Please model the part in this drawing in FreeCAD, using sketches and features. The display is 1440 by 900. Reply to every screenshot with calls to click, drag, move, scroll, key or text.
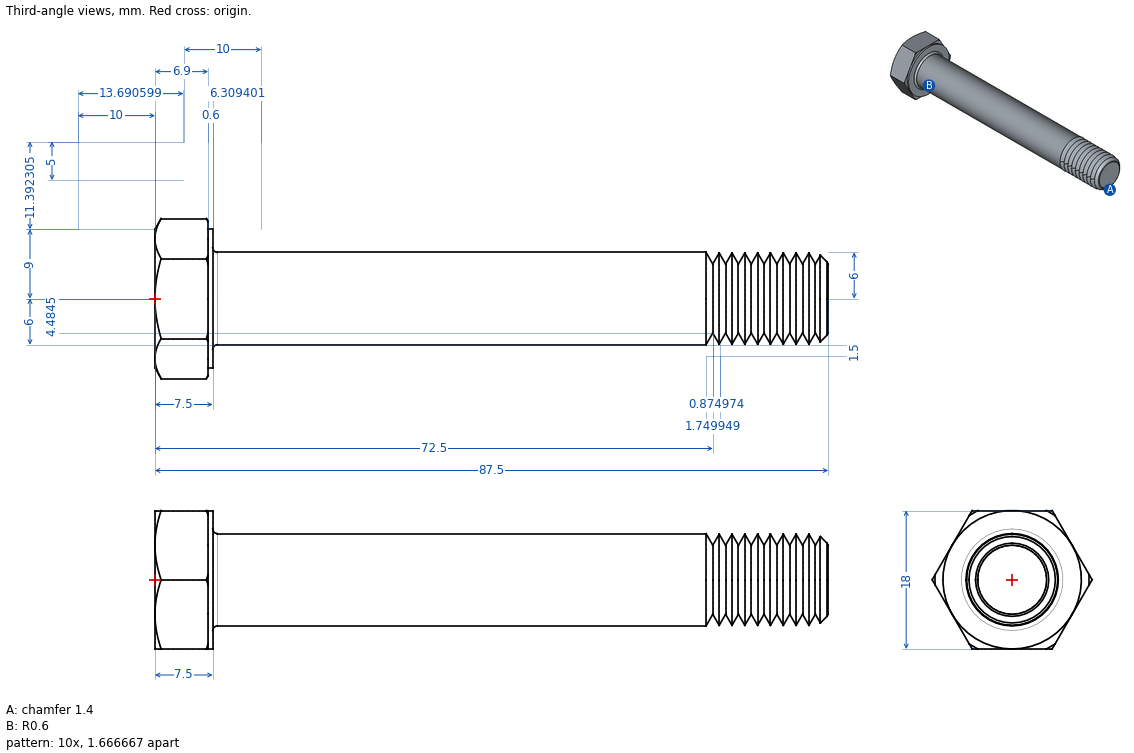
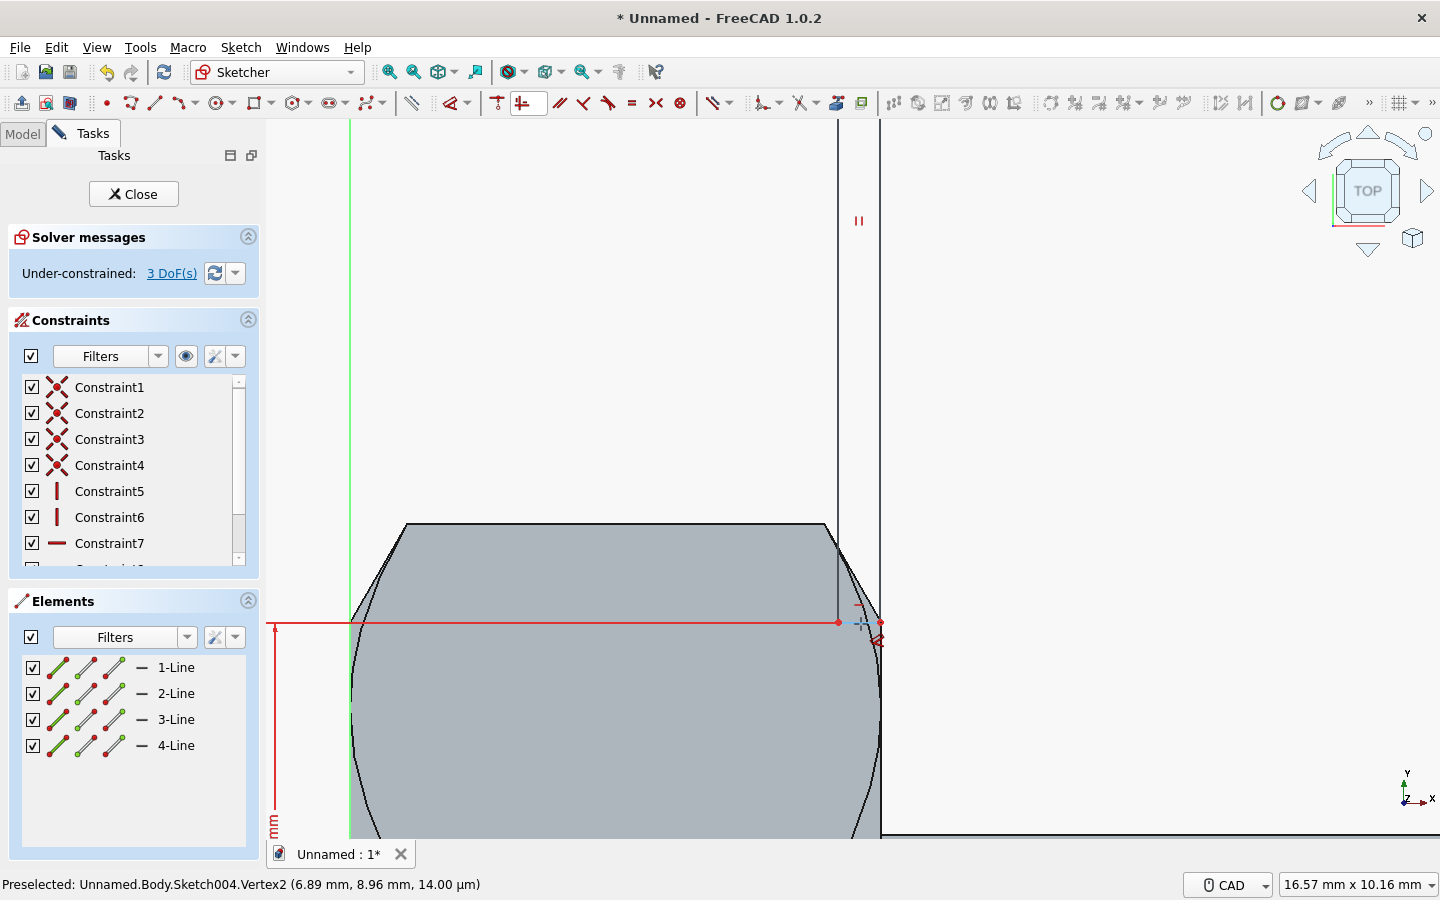
click(859, 623)
click(859, 657)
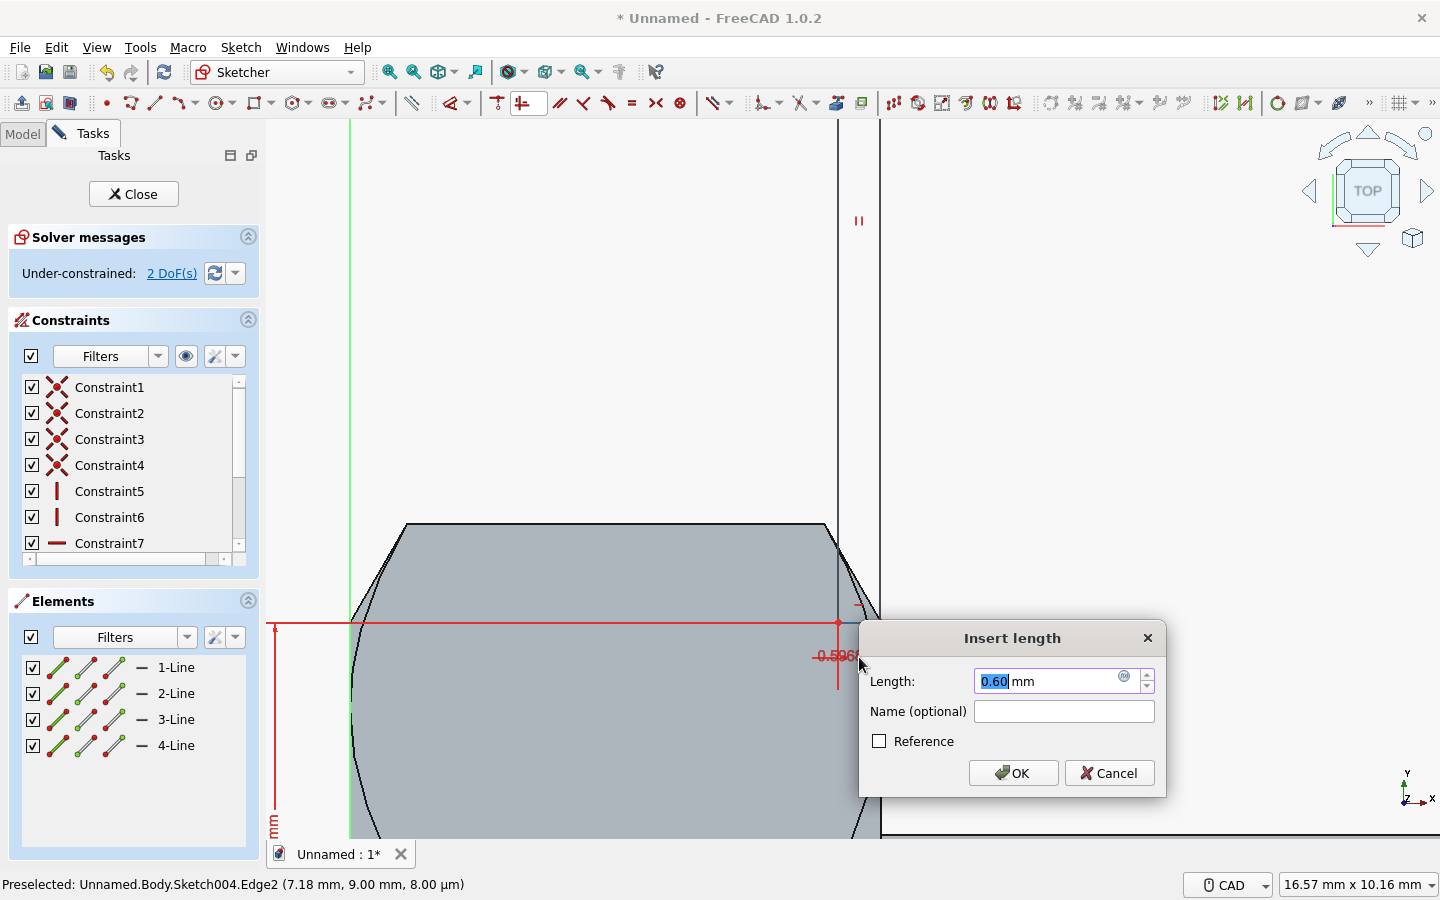
text(0.6)
key(Return)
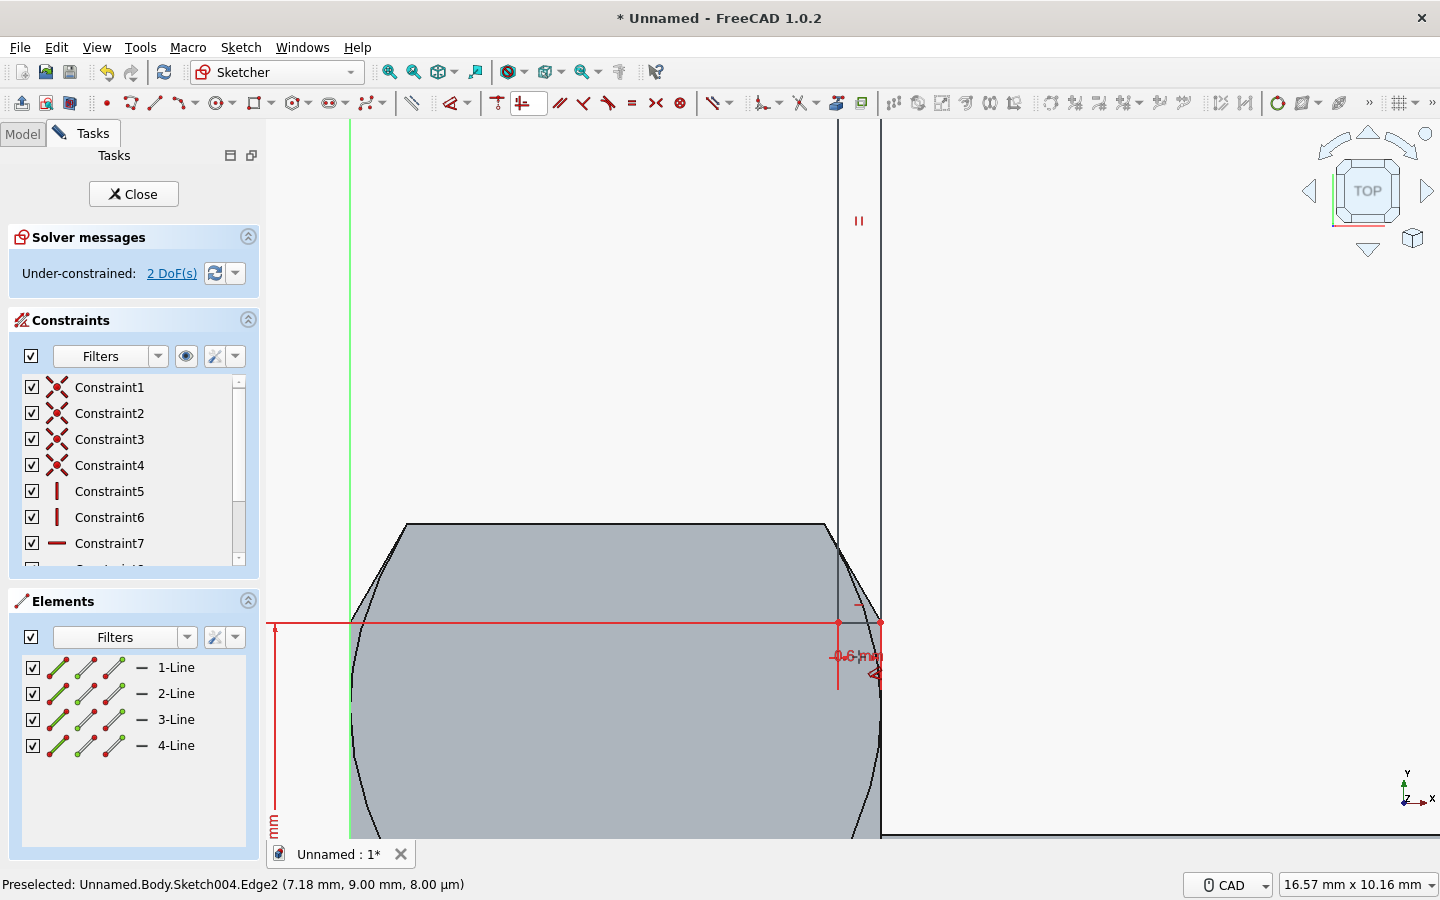
scroll(857, 454, down, 6)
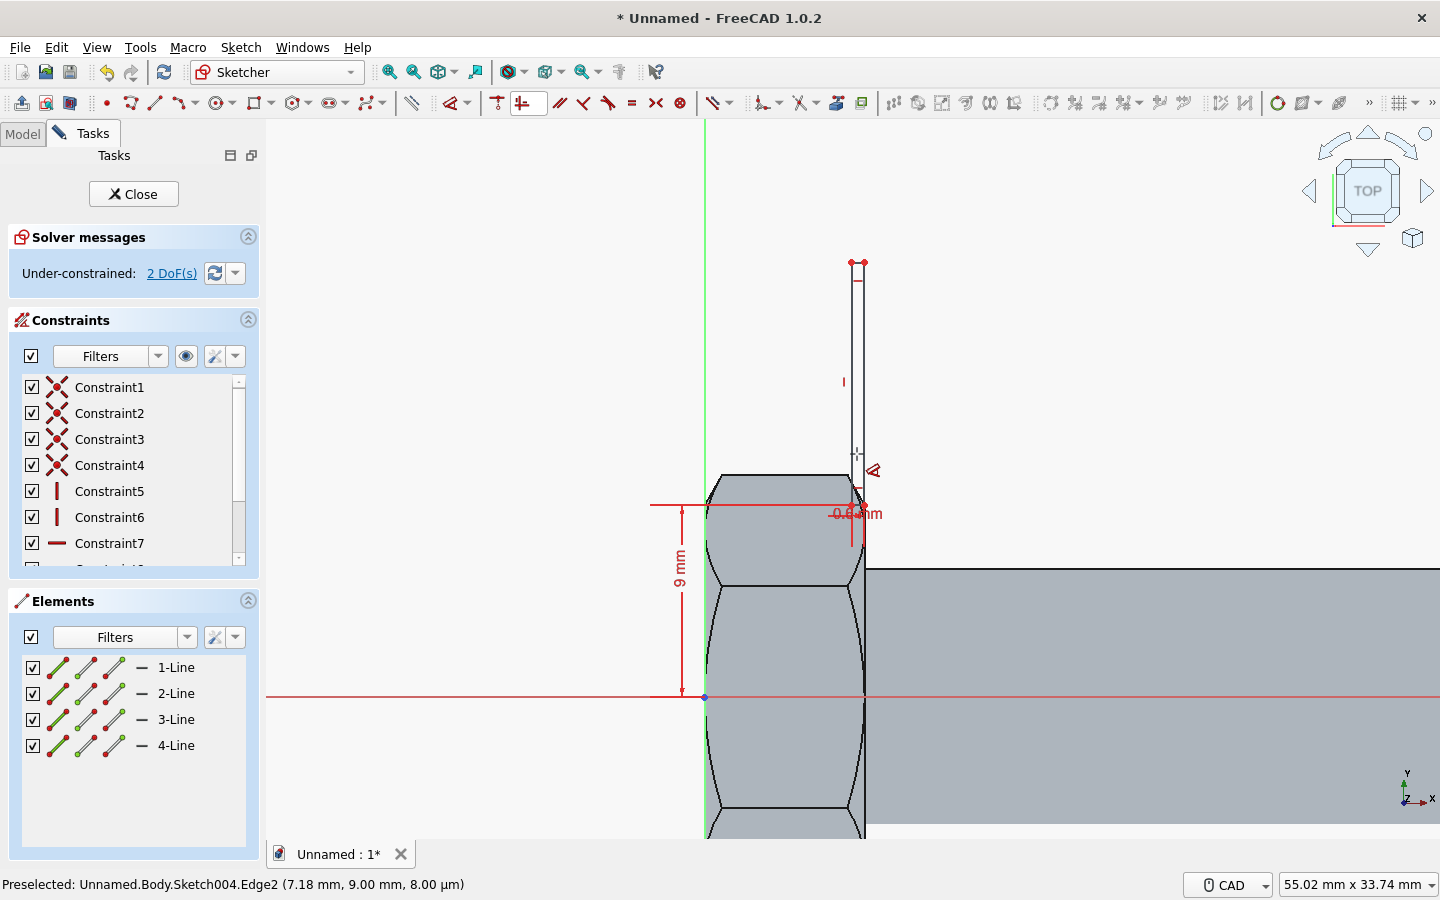
click(852, 263)
click(778, 731)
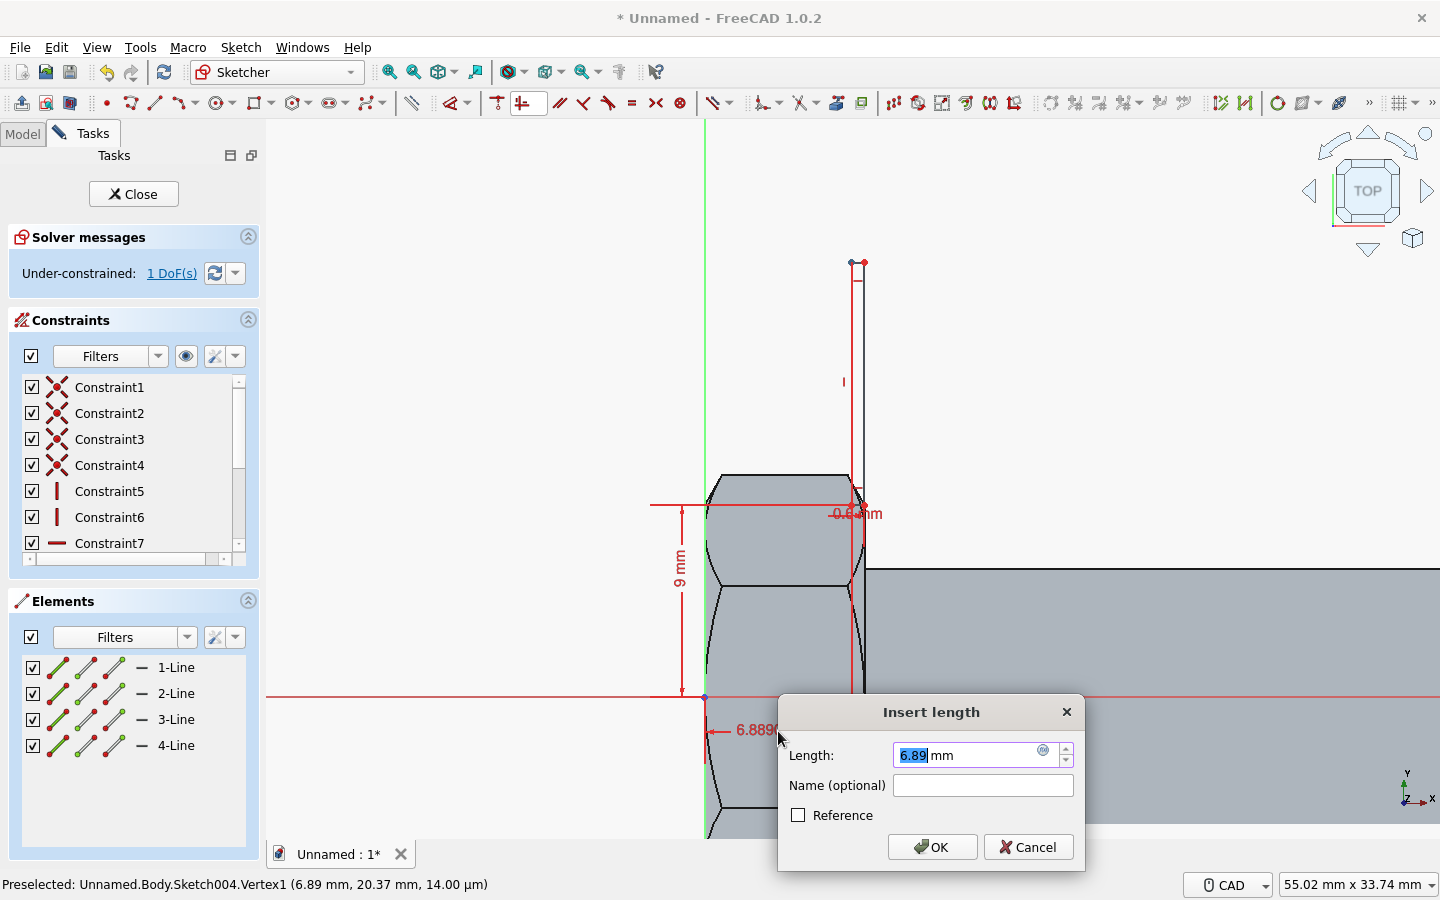
text(6.9)
key(Return)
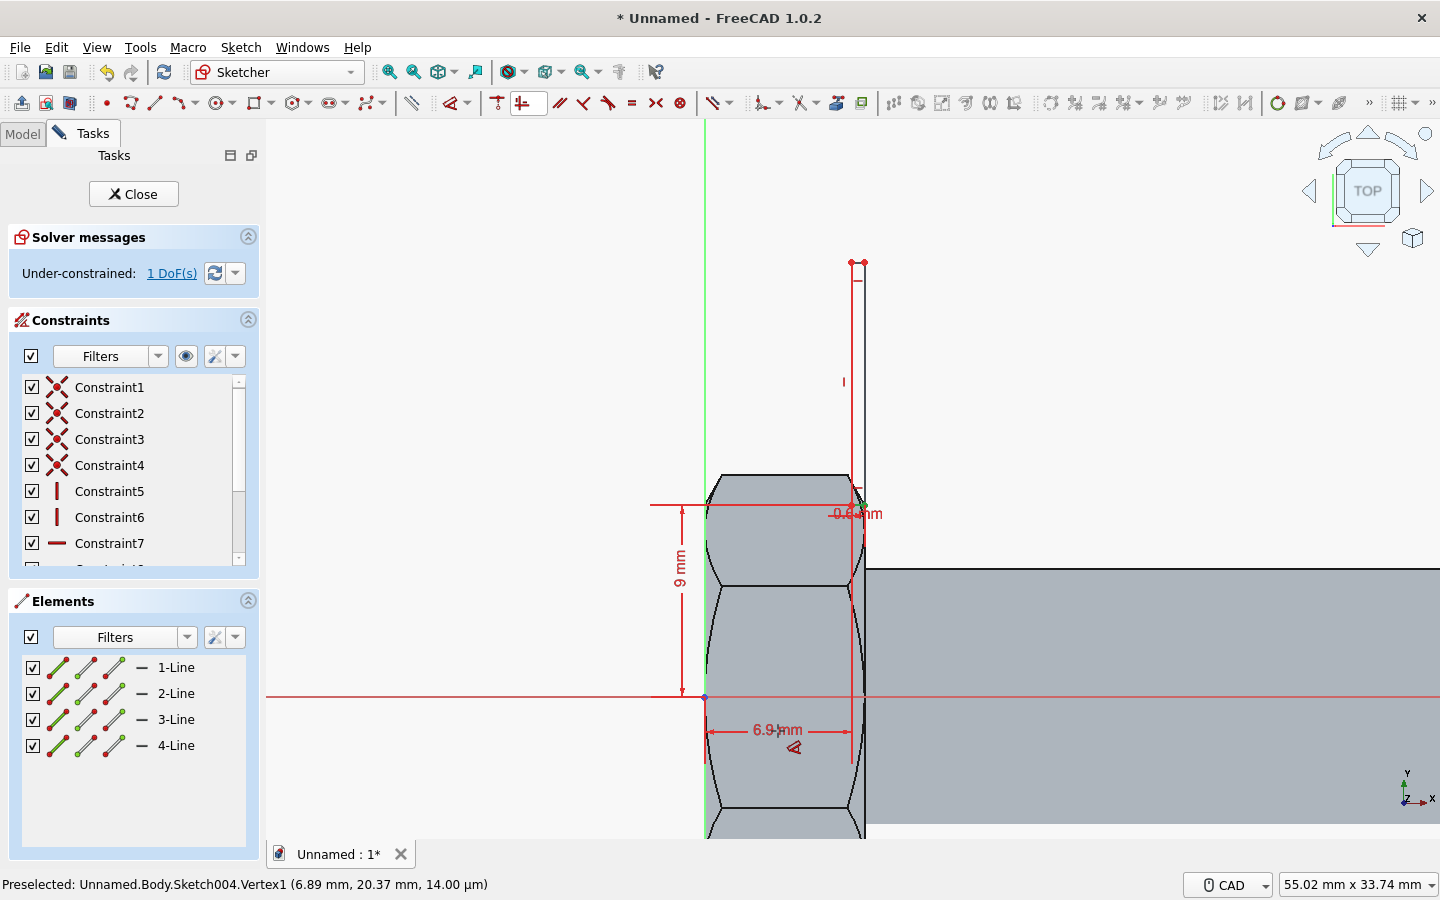
click(852, 335)
click(886, 384)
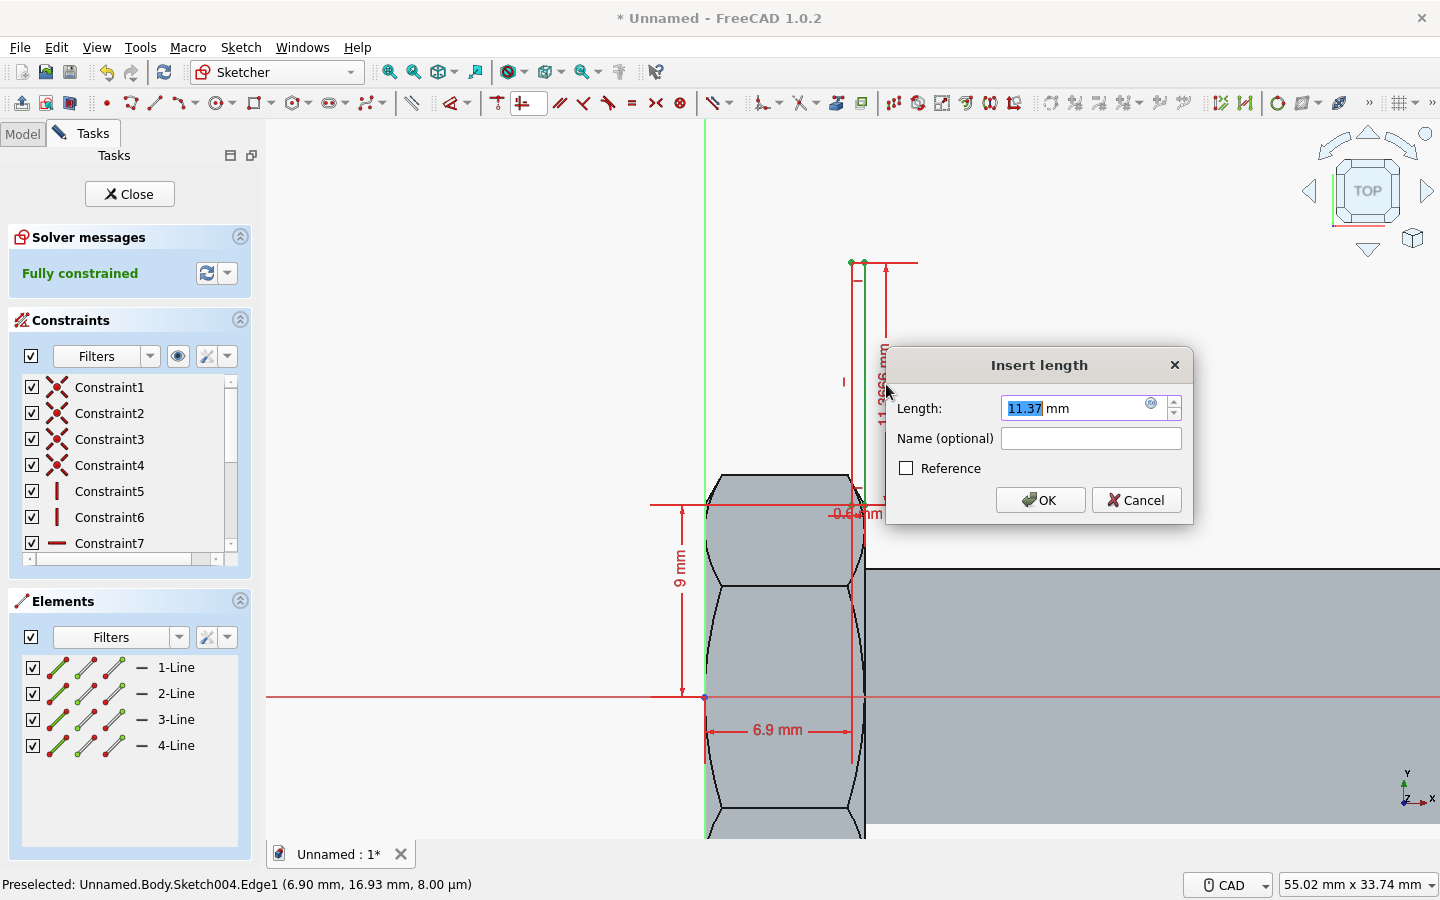
text(11.392305)
key(Return)
key(Escape)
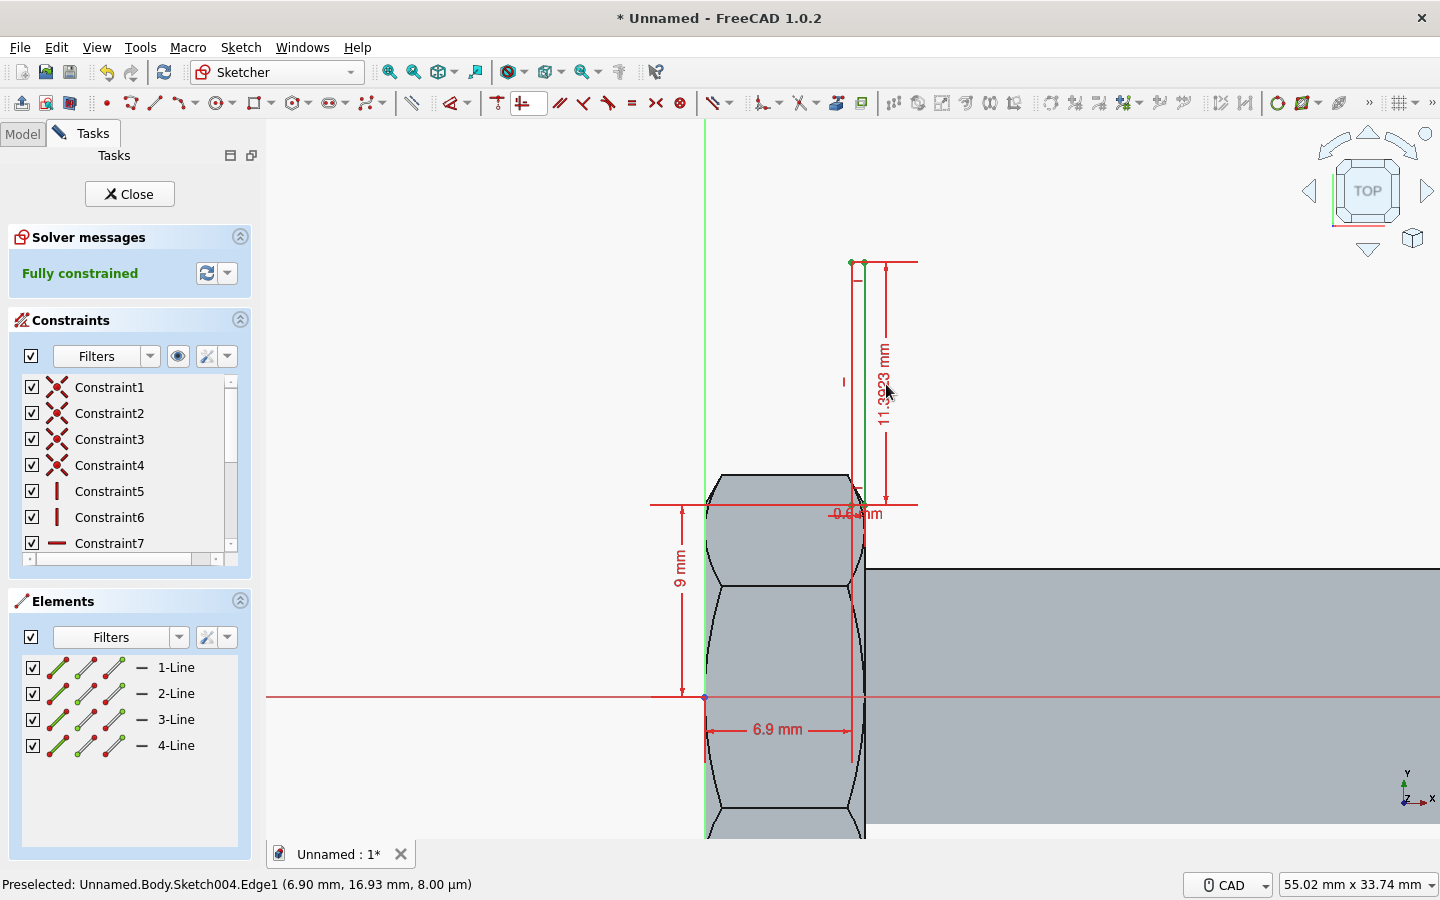
click(130, 194)